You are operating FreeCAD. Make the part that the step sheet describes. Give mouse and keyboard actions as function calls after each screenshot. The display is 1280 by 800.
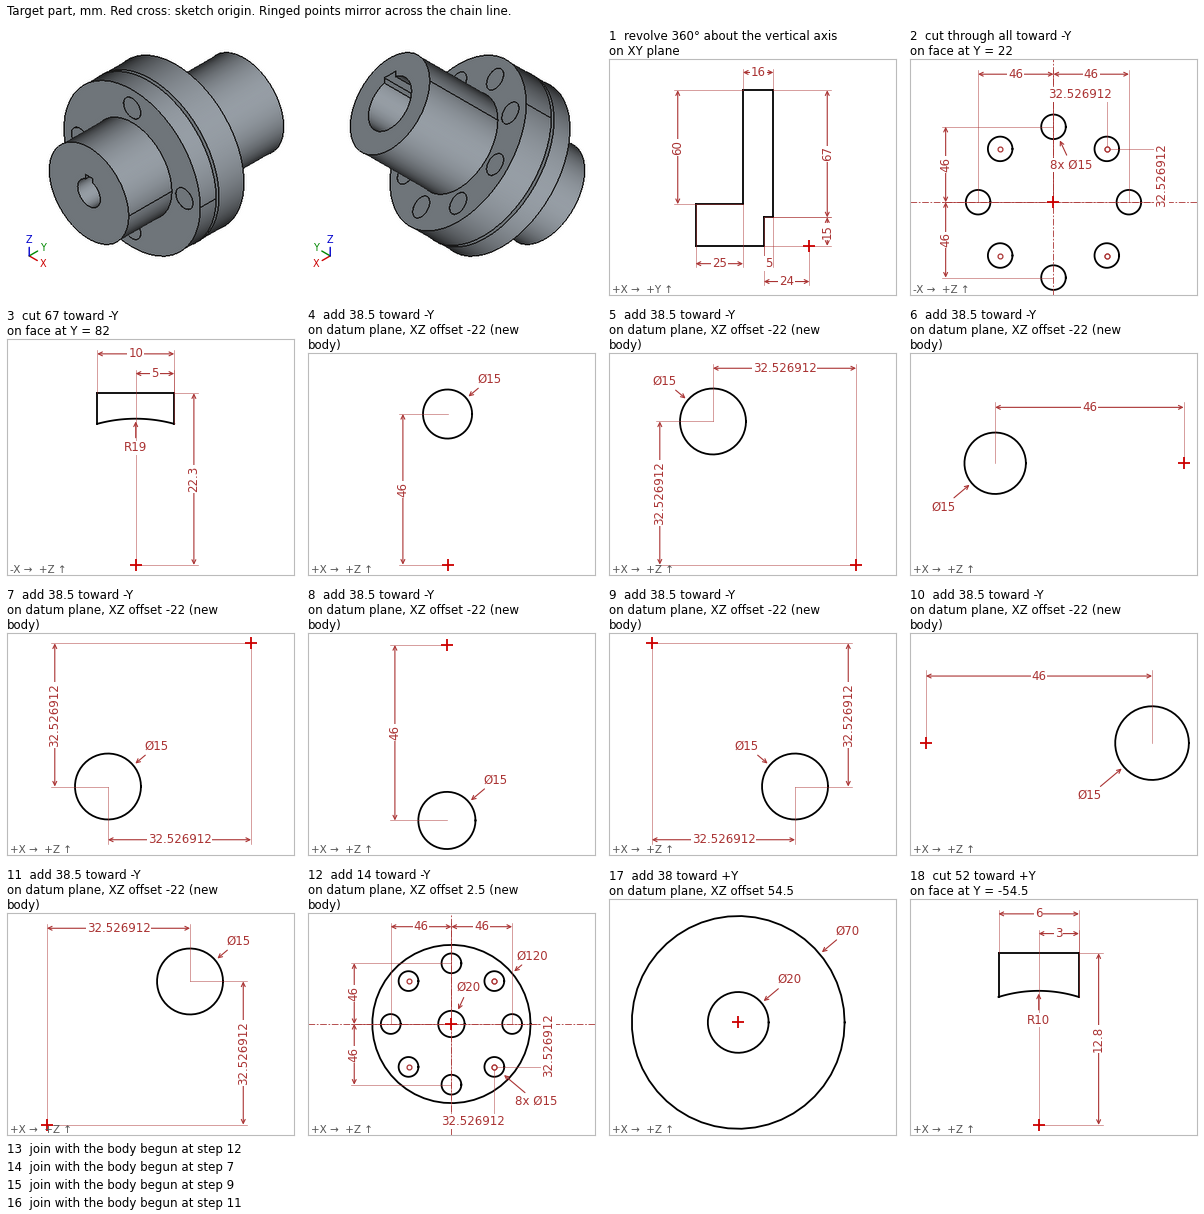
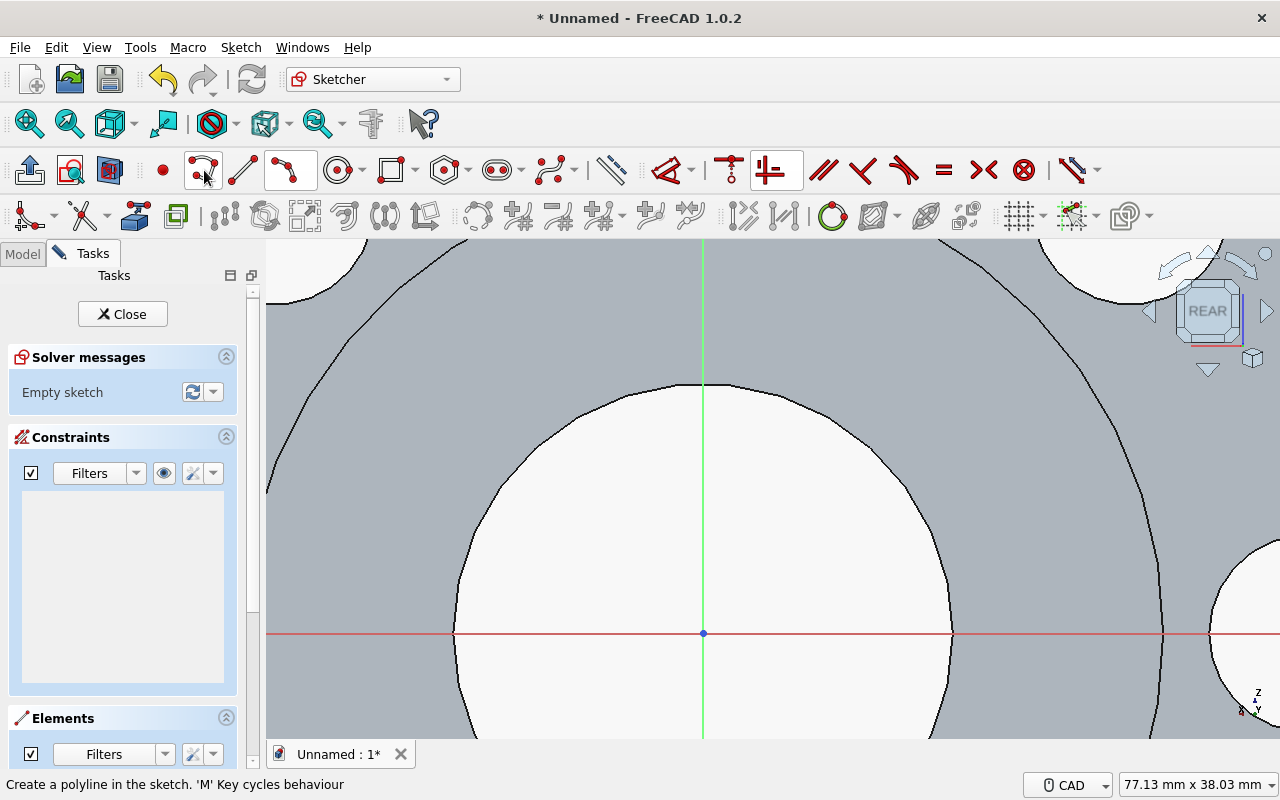
click(769, 393)
click(769, 340)
click(637, 340)
click(637, 393)
right_click(637, 393)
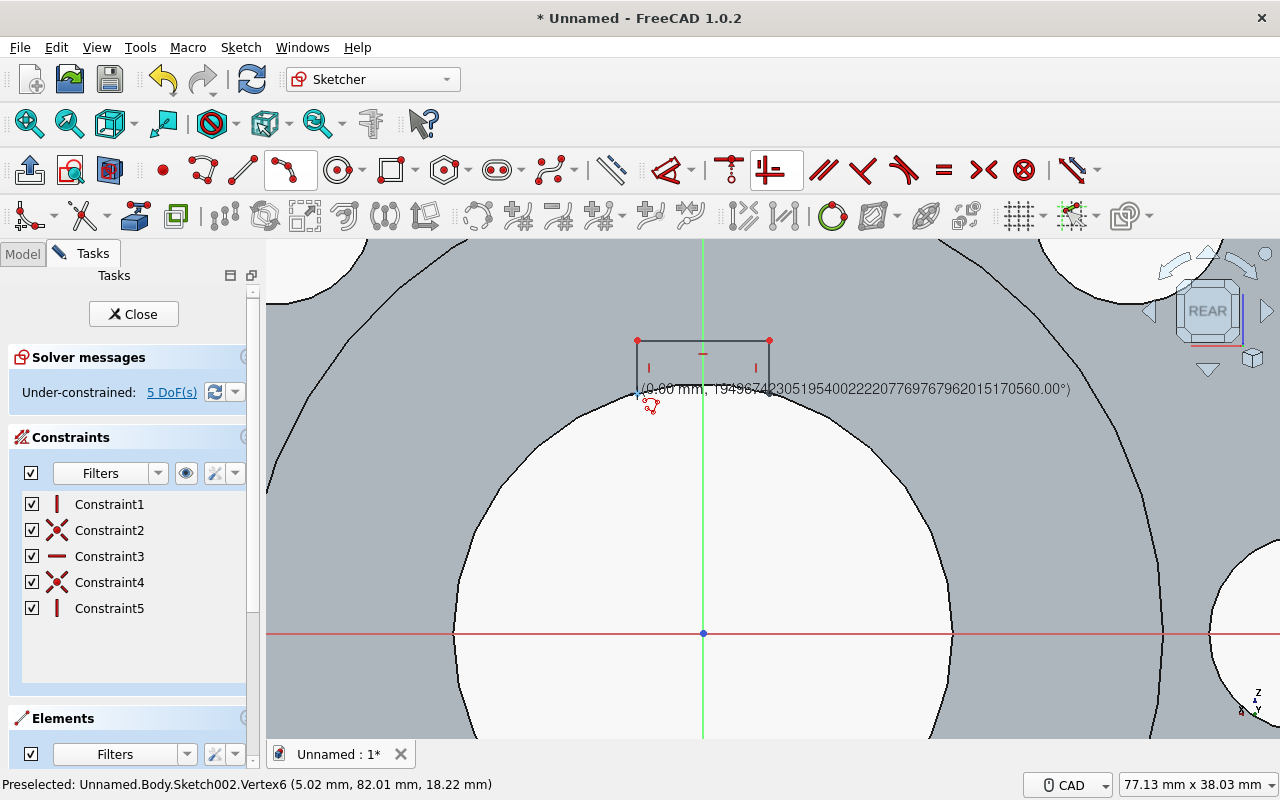
click(284, 170)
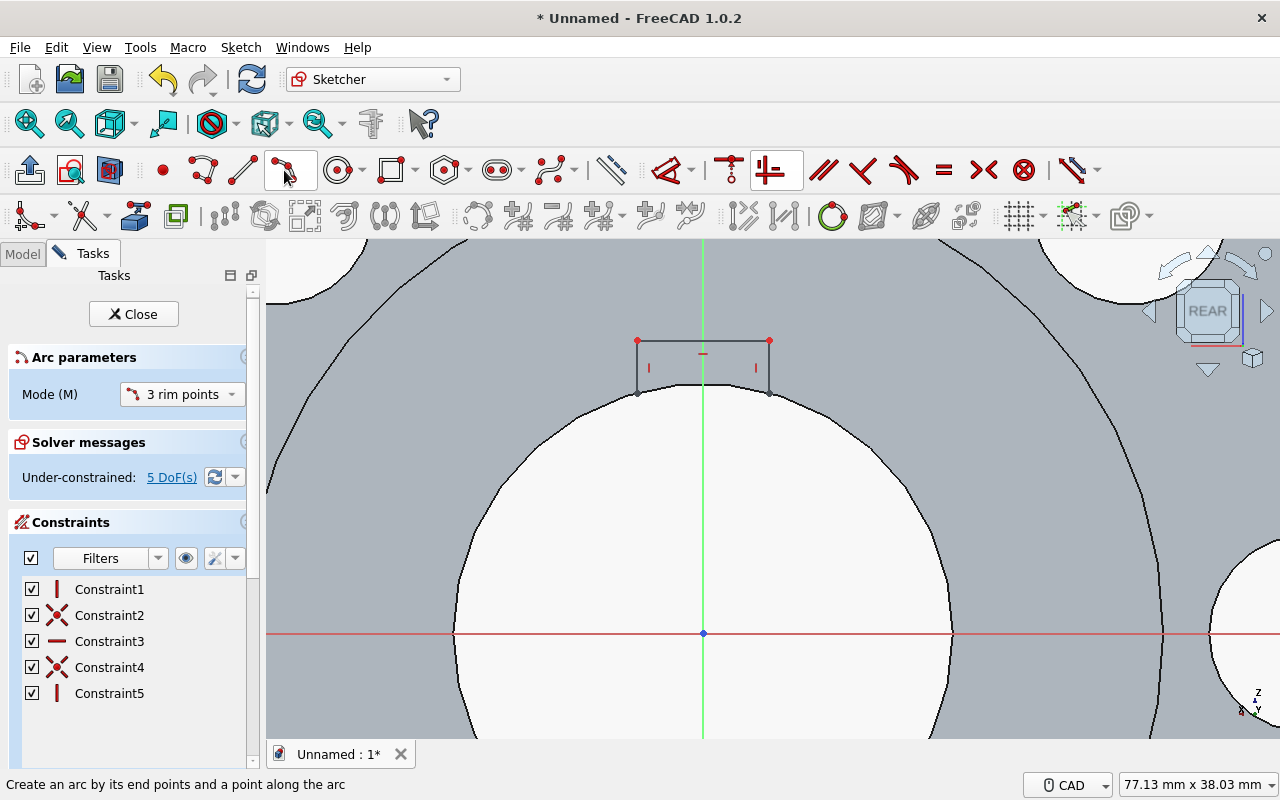
click(637, 394)
click(769, 394)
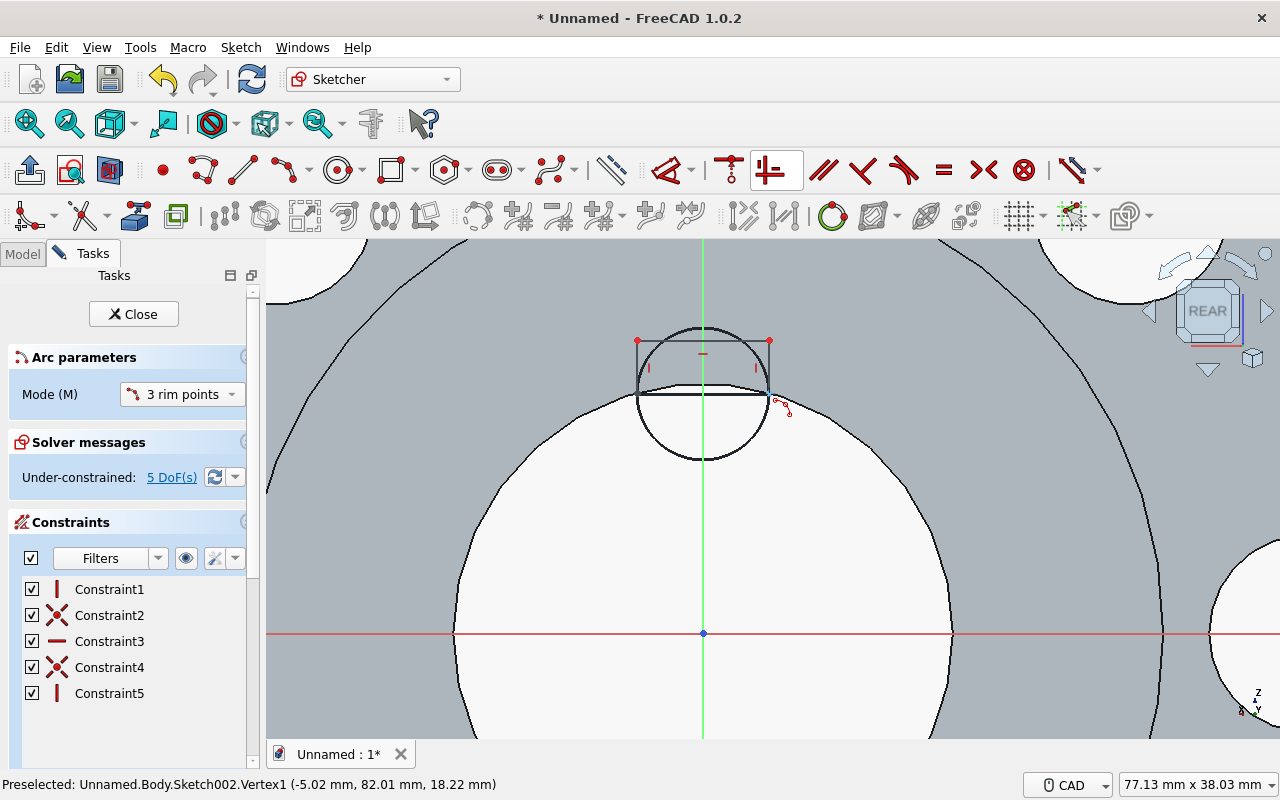
scroll(716, 384, up, 4)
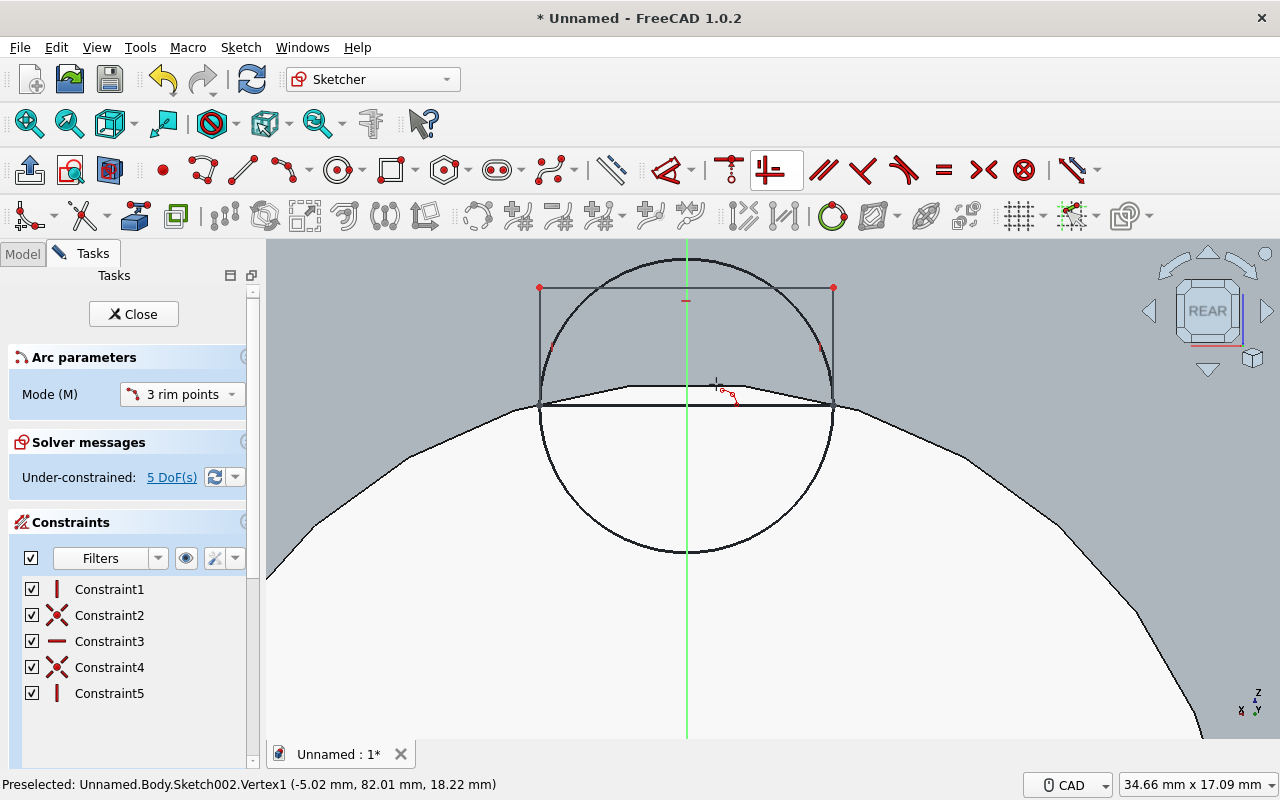
click(716, 384)
key(Escape)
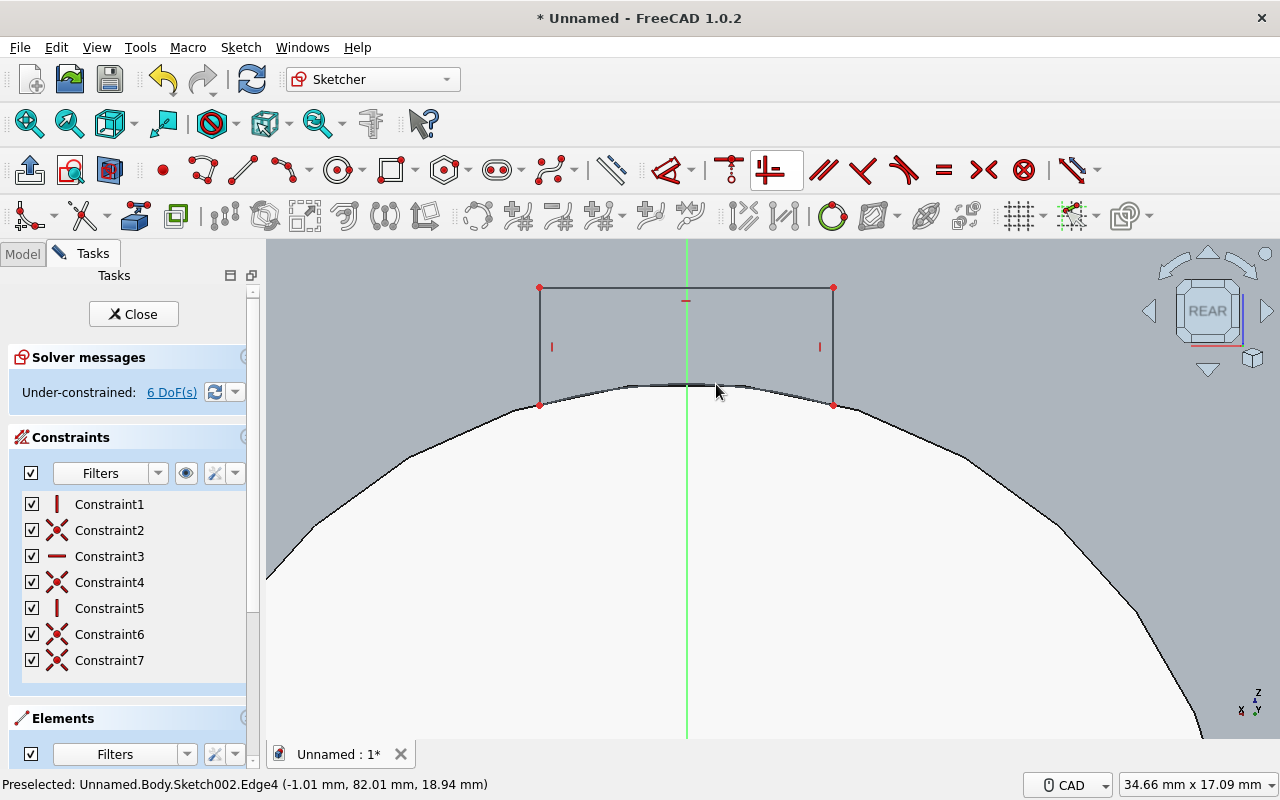
scroll(719, 388, down, 4)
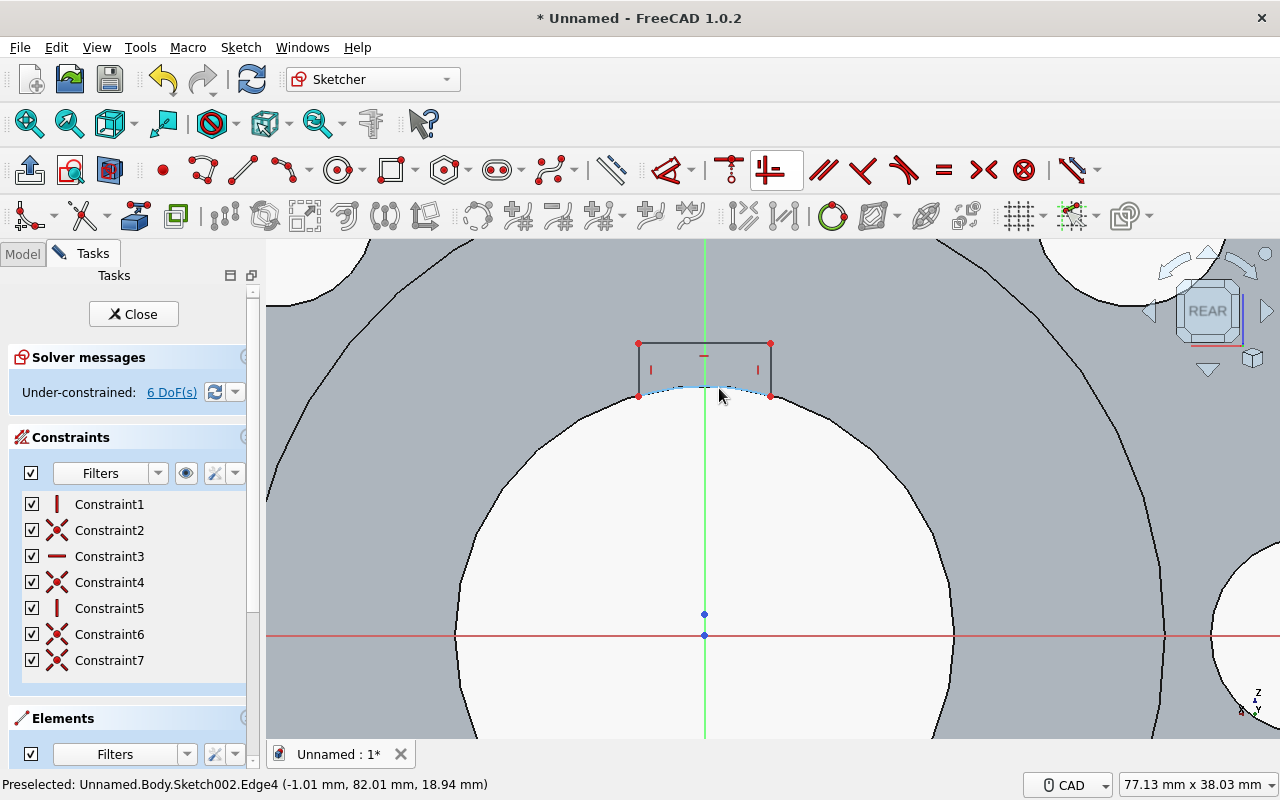
drag(695, 604, 715, 646)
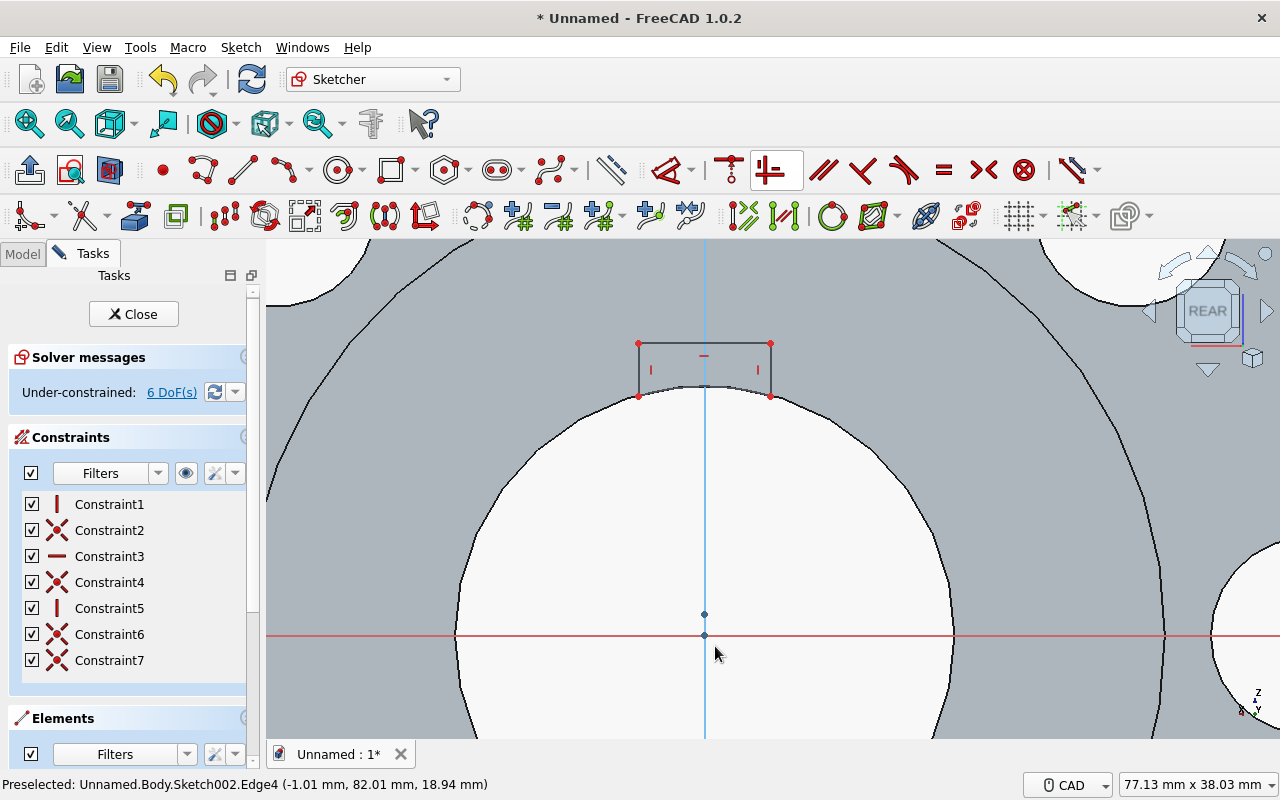
click(730, 170)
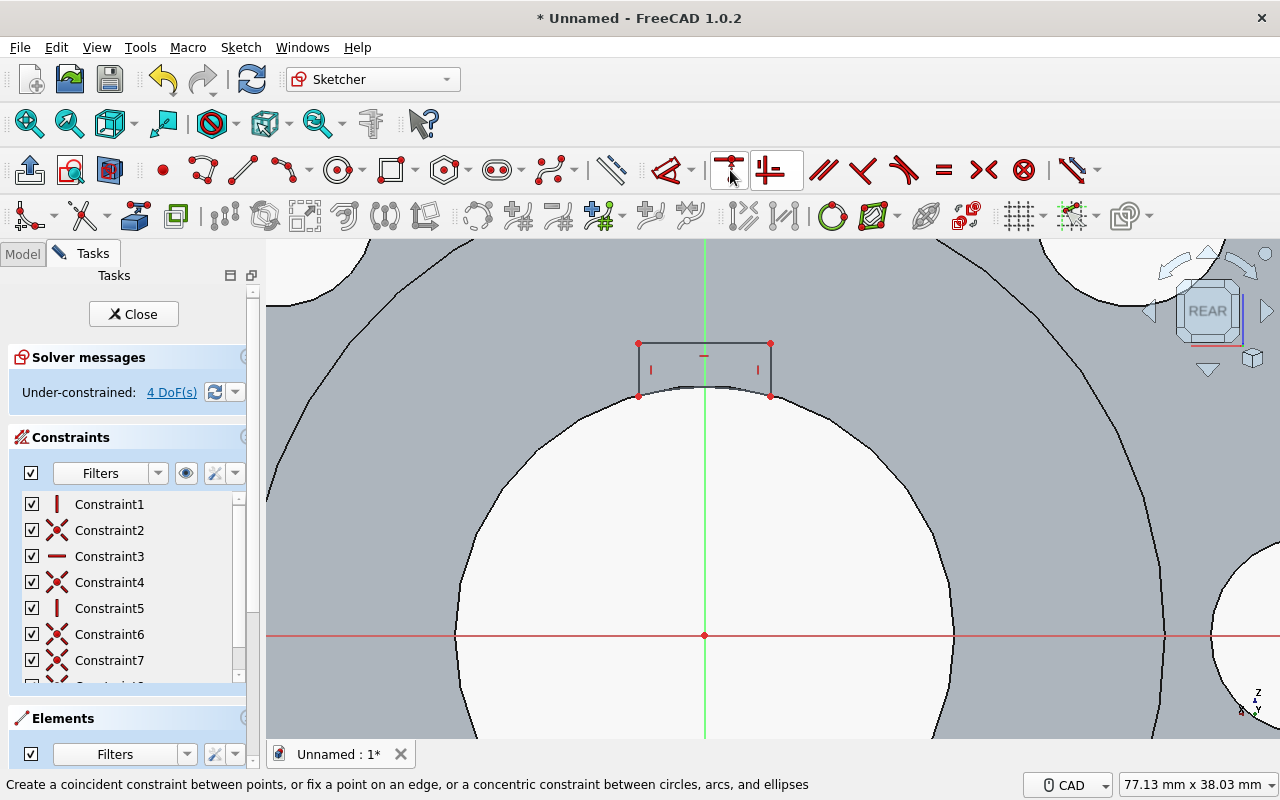
click(666, 170)